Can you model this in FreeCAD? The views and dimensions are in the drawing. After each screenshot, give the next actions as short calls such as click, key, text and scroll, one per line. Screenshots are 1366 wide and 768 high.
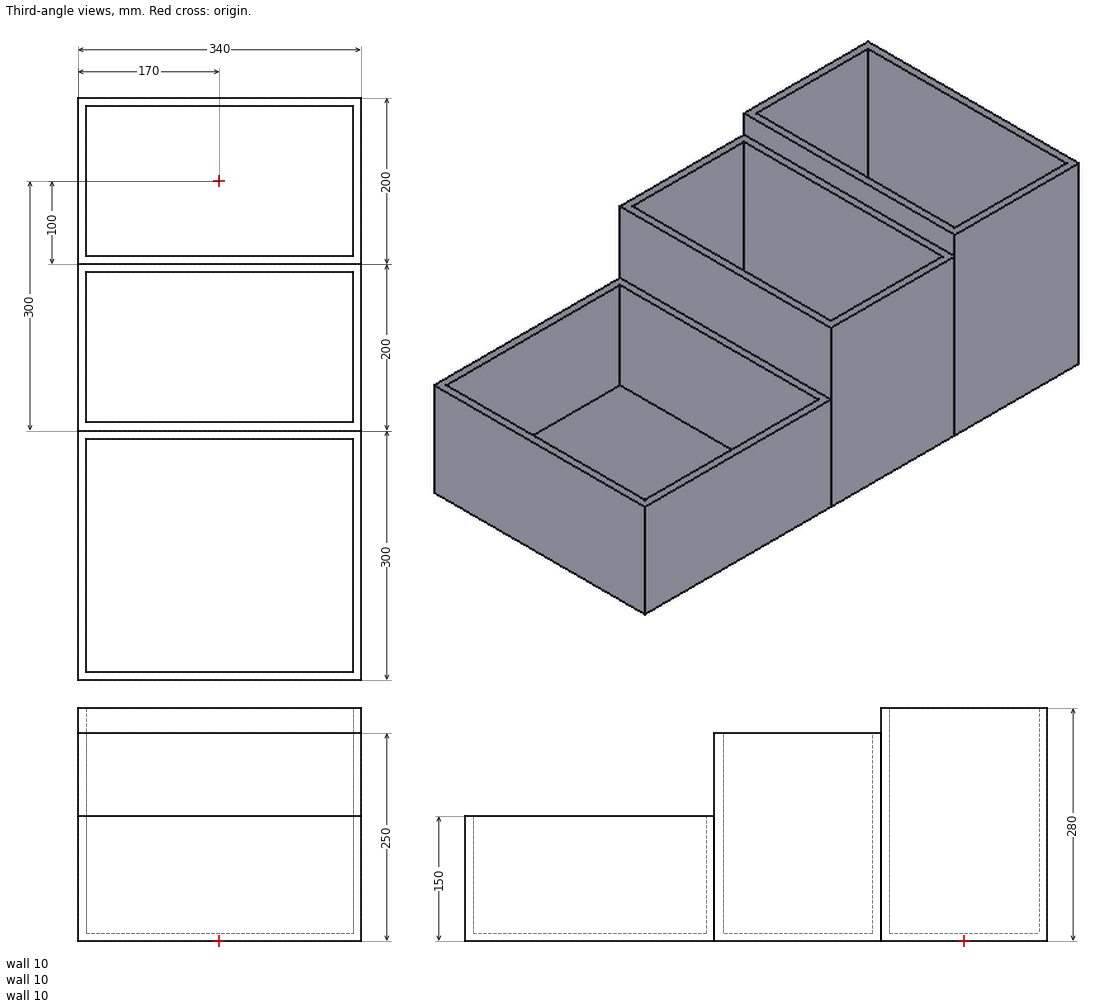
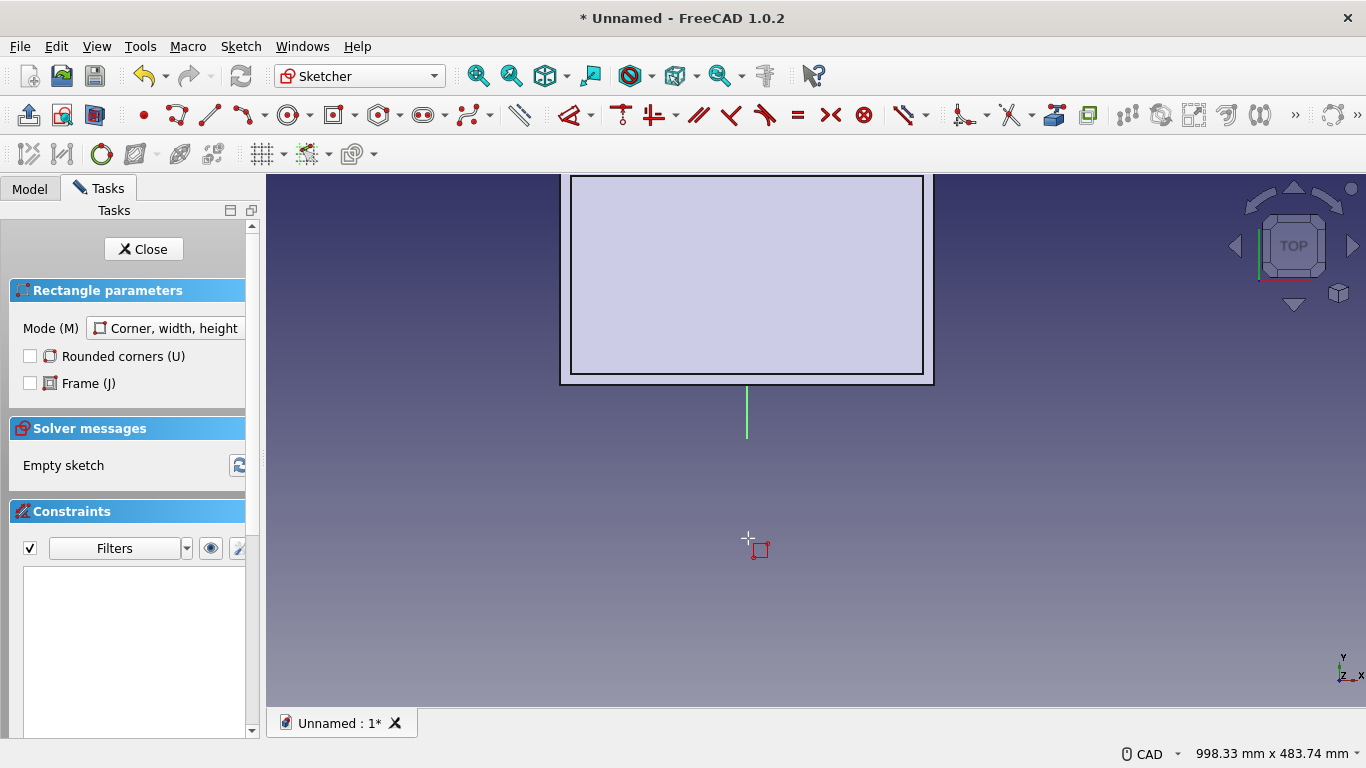
click(560, 385)
move(934, 605)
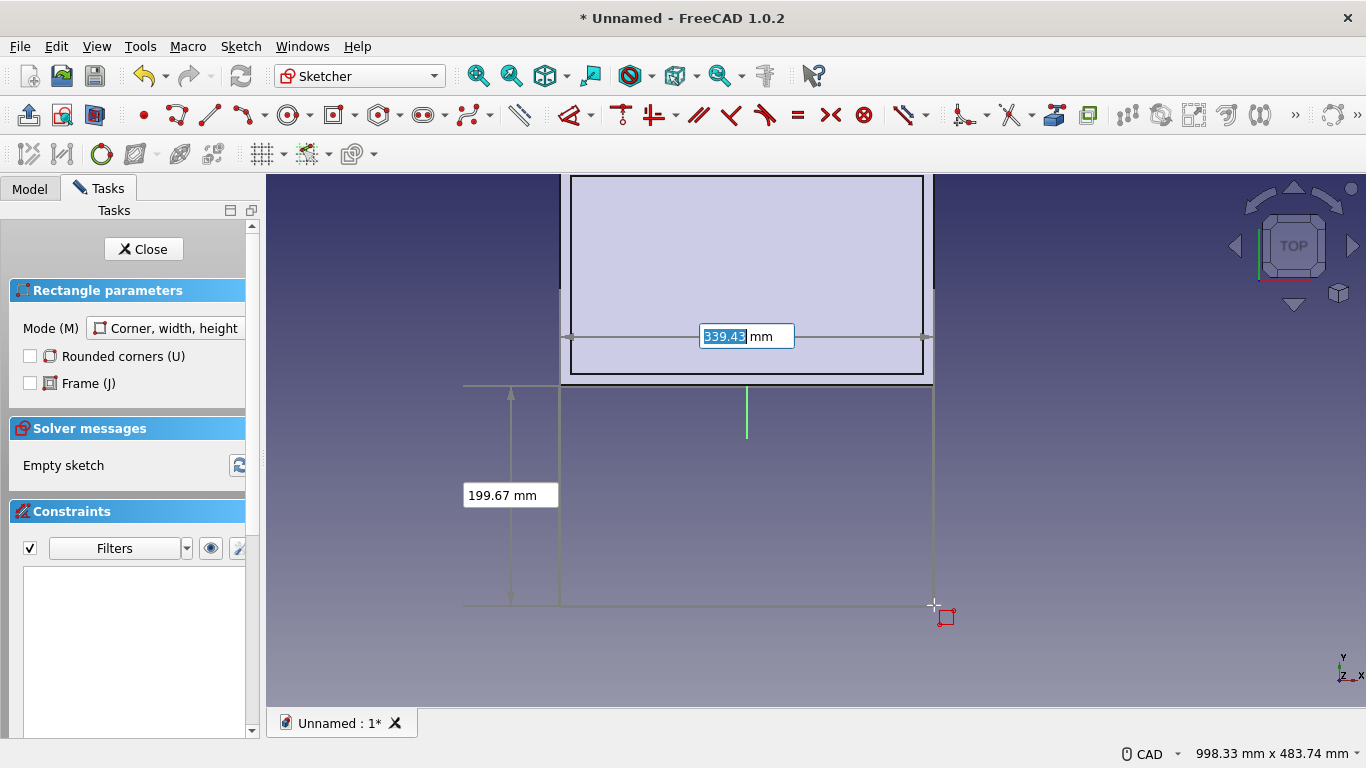
text(340)
key(Tab)
text(200)
key(Return)
key(Escape)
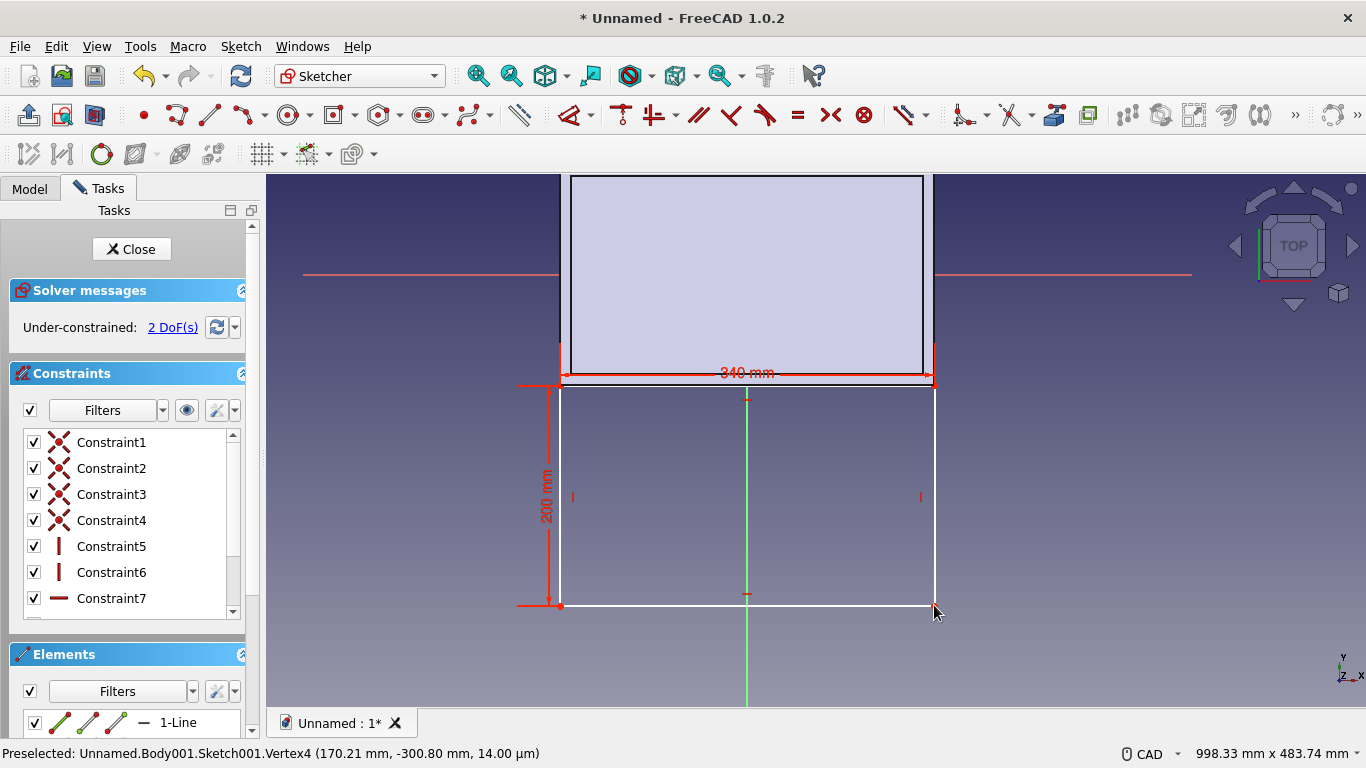
click(568, 116)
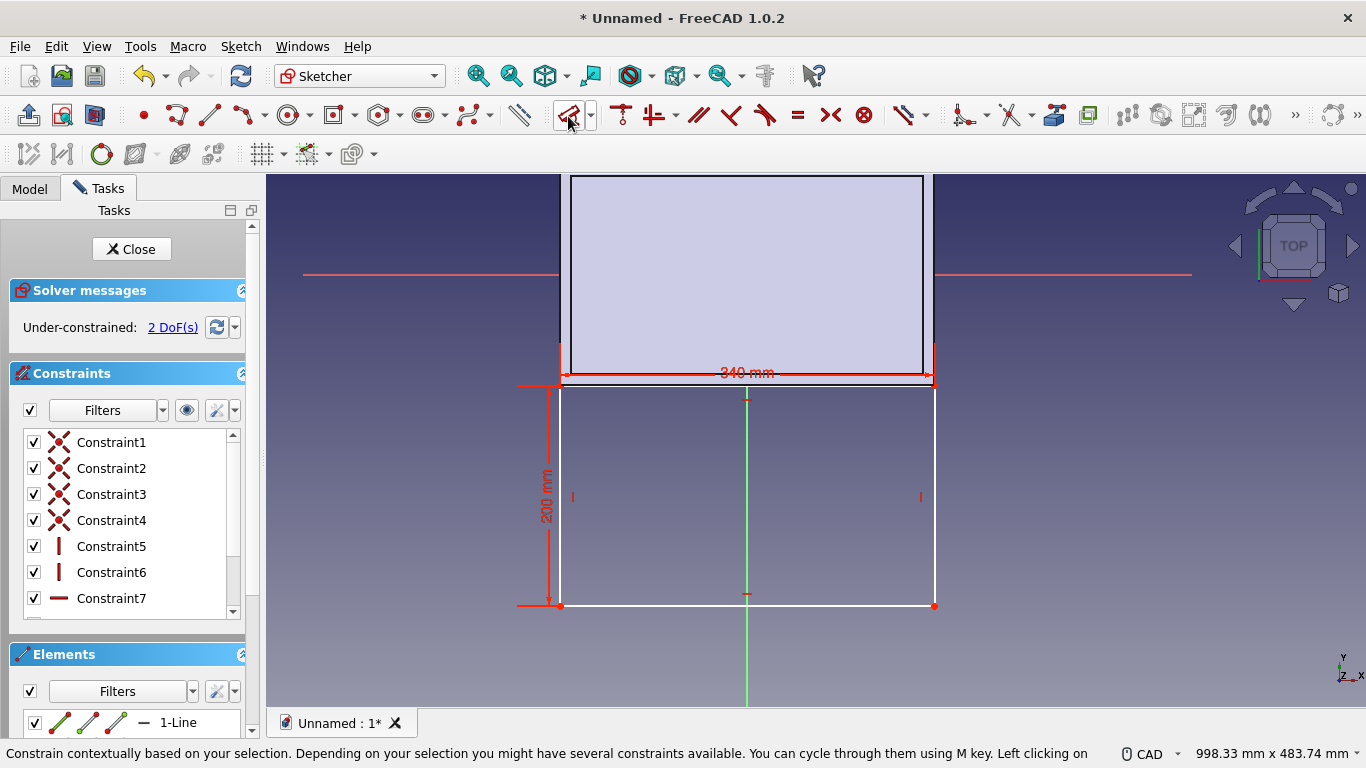
click(560, 386)
click(654, 241)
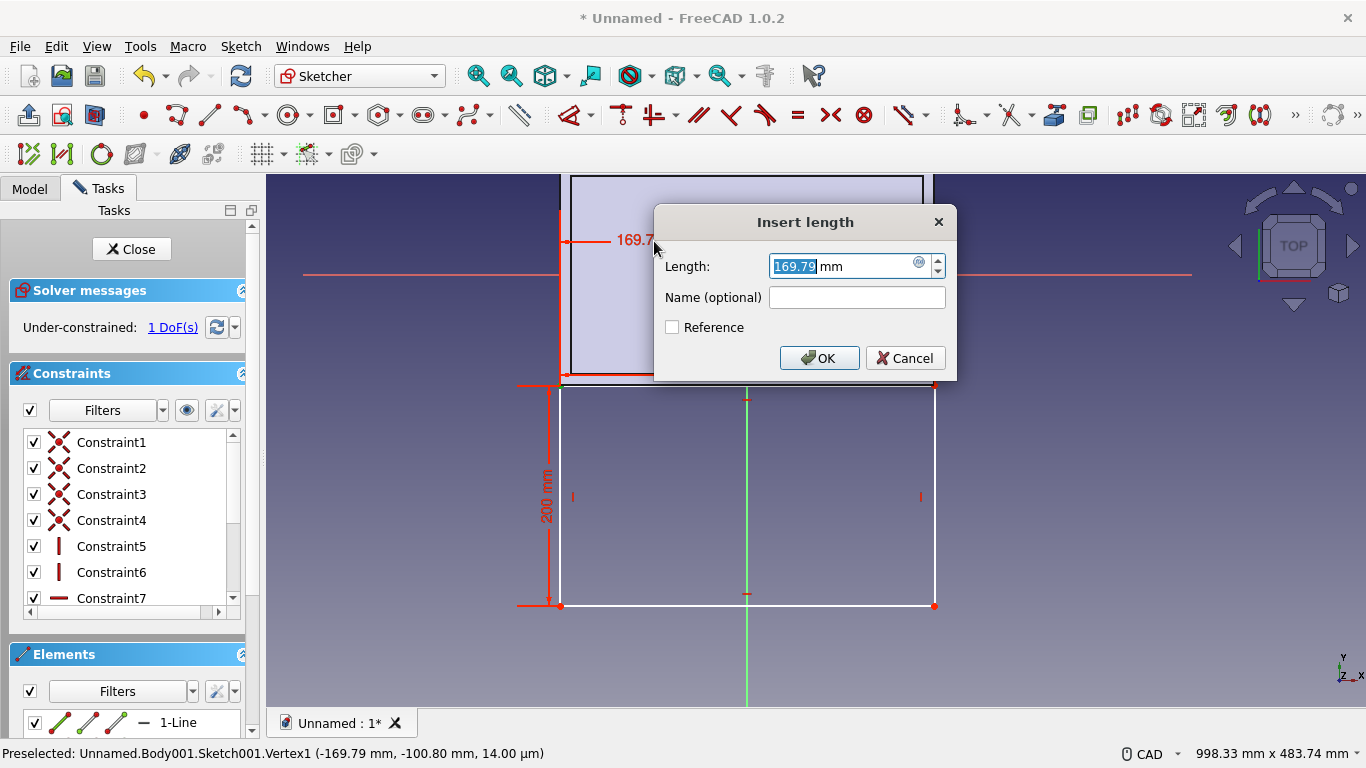
text(170)
key(Return)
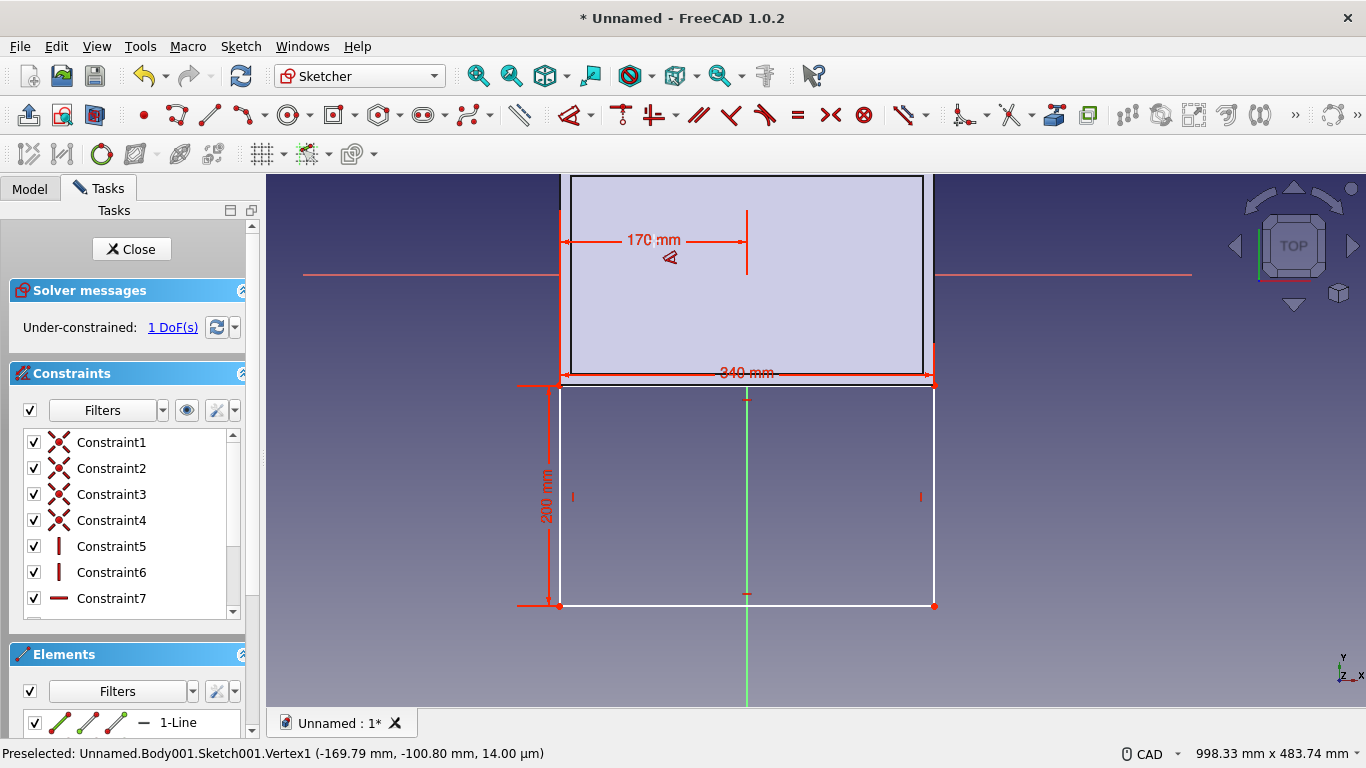
click(560, 386)
click(526, 330)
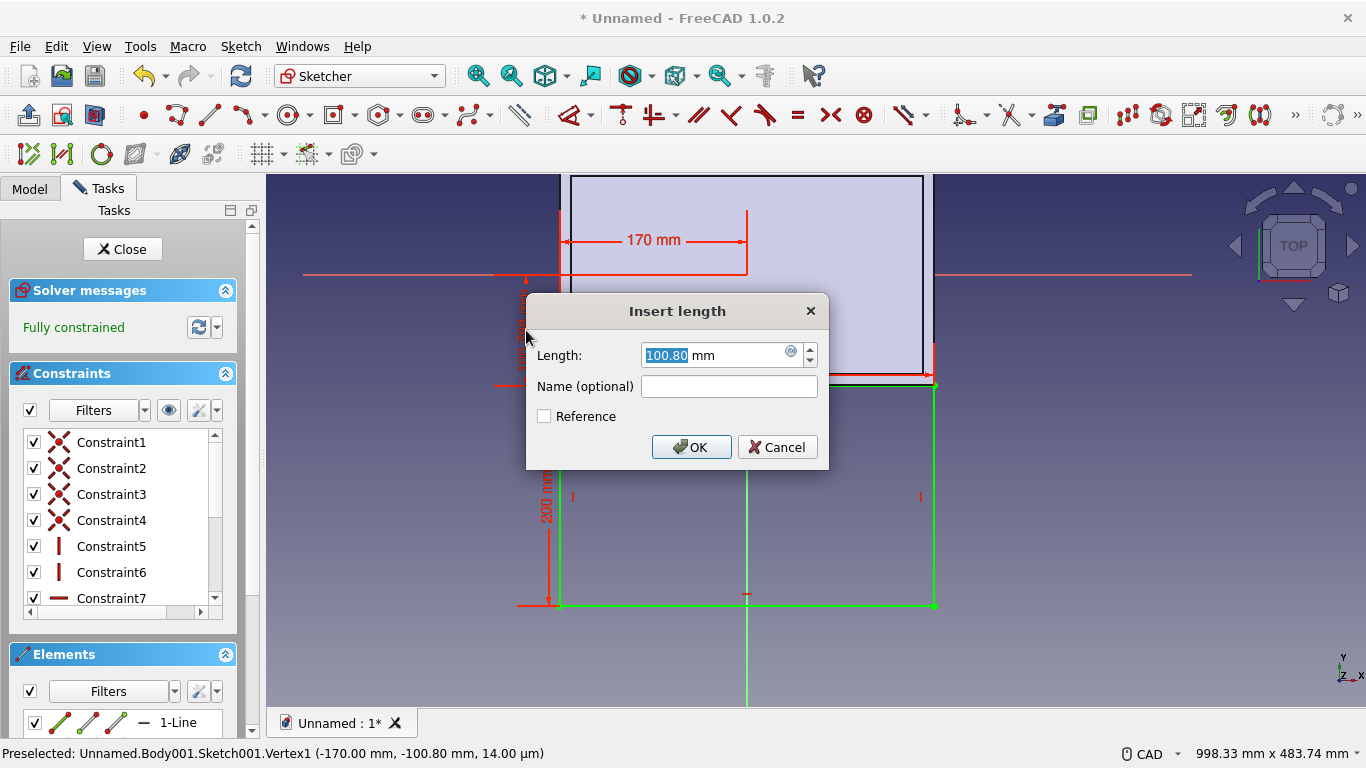
text(100)
key(Return)
key(Escape)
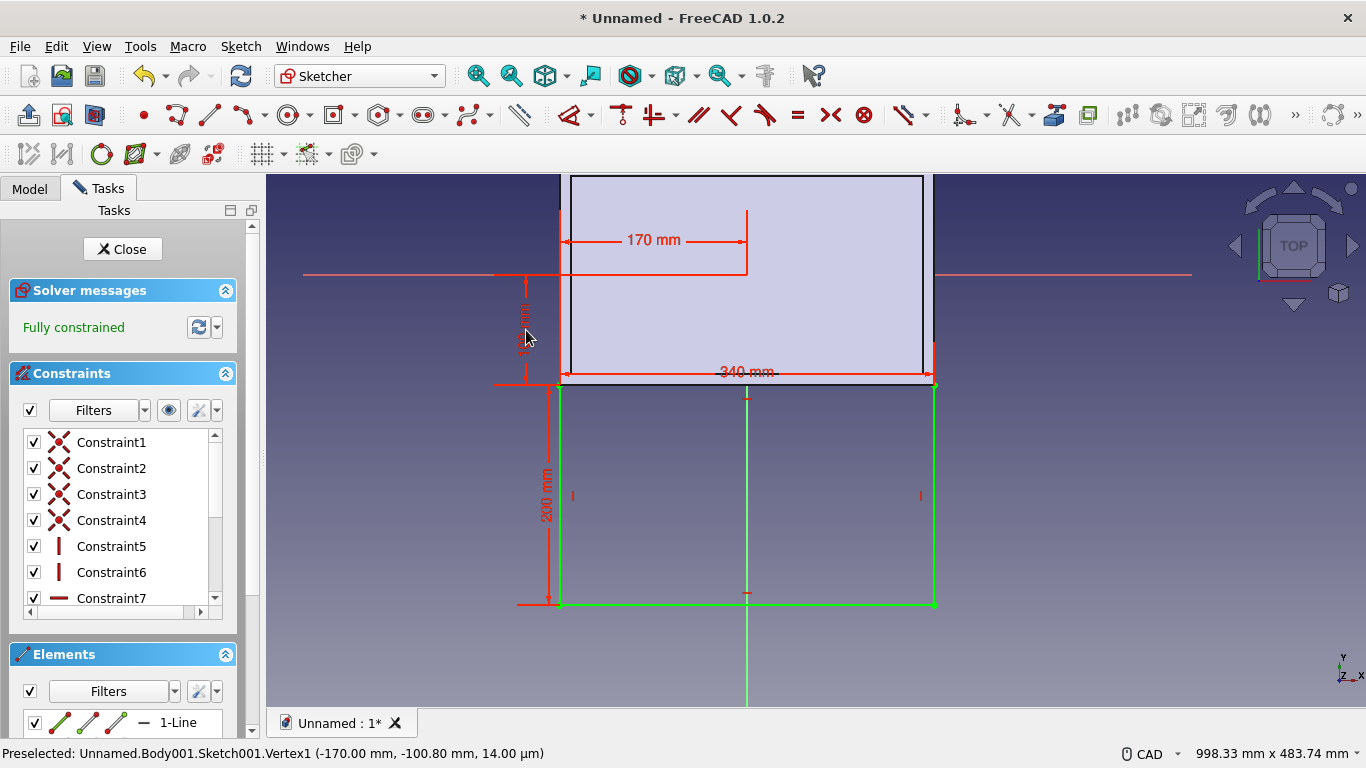
click(123, 249)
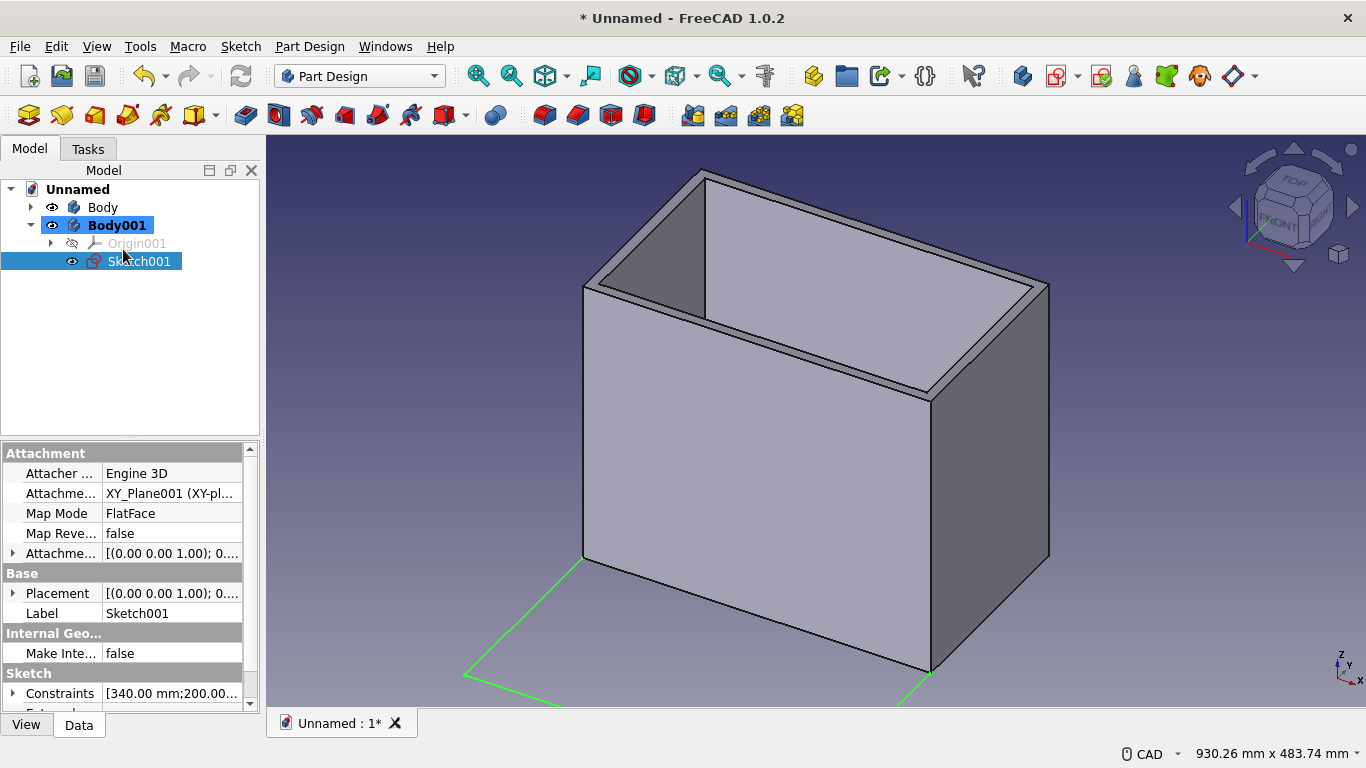
click(29, 116)